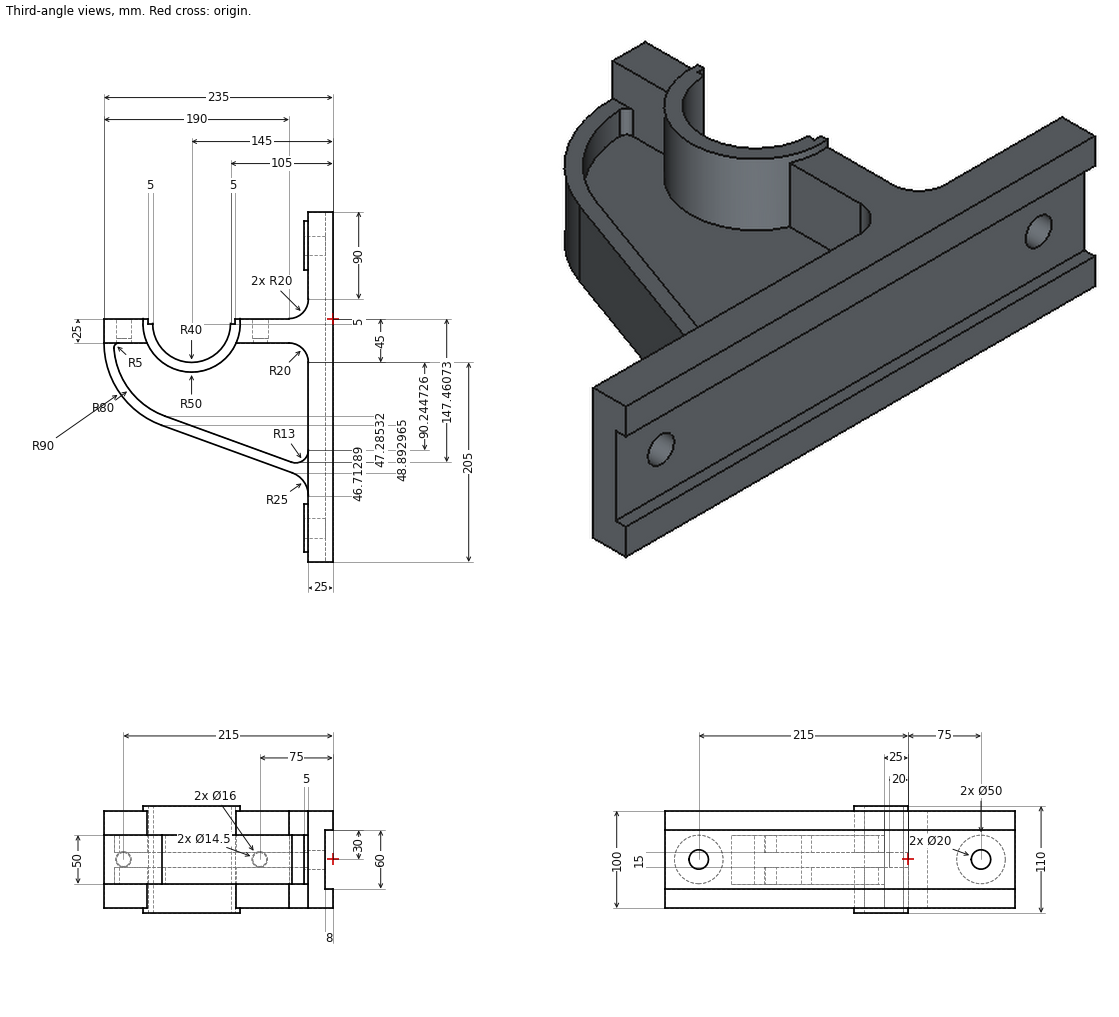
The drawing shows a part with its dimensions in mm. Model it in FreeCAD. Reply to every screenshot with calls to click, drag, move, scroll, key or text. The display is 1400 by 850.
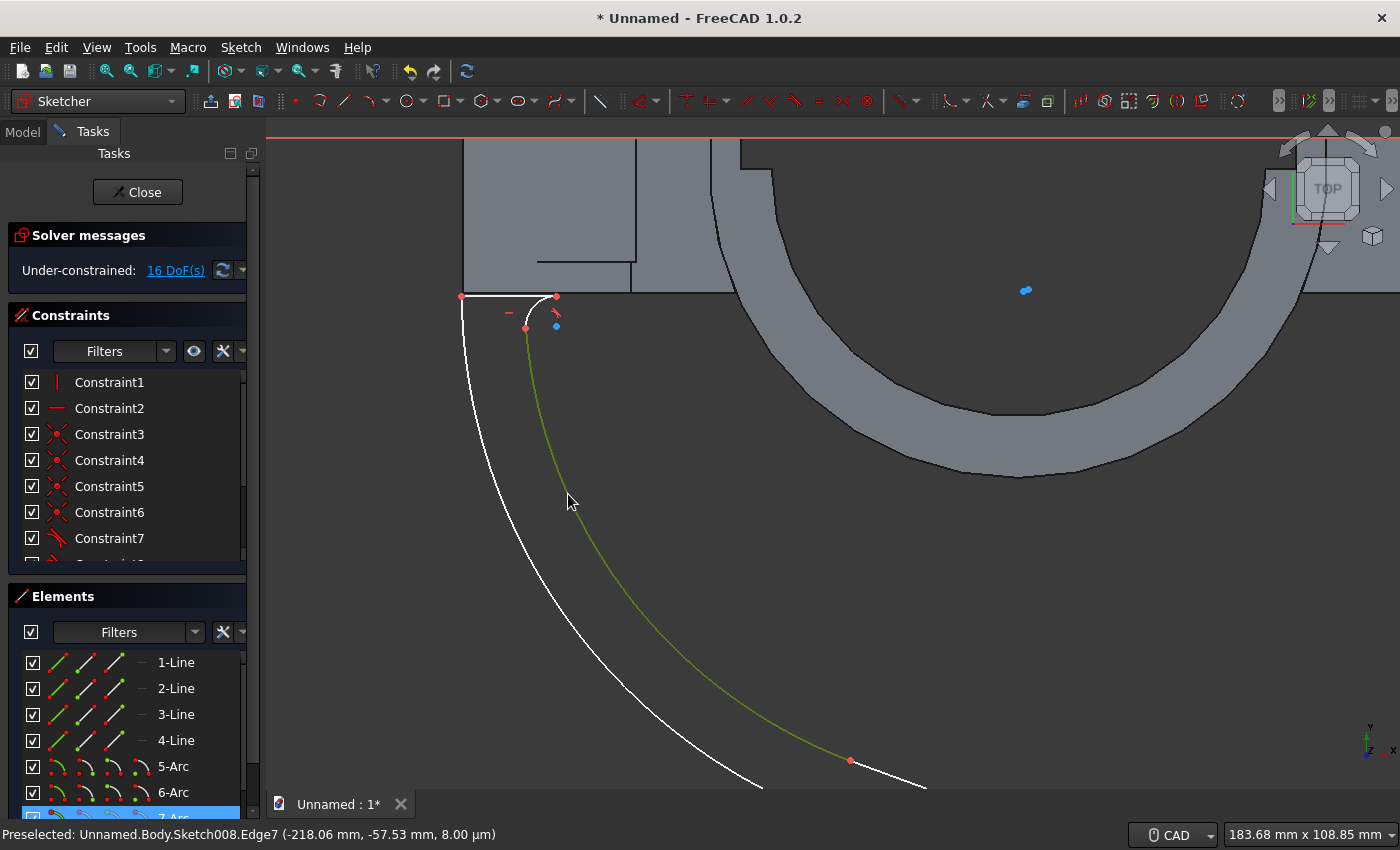
click(529, 314)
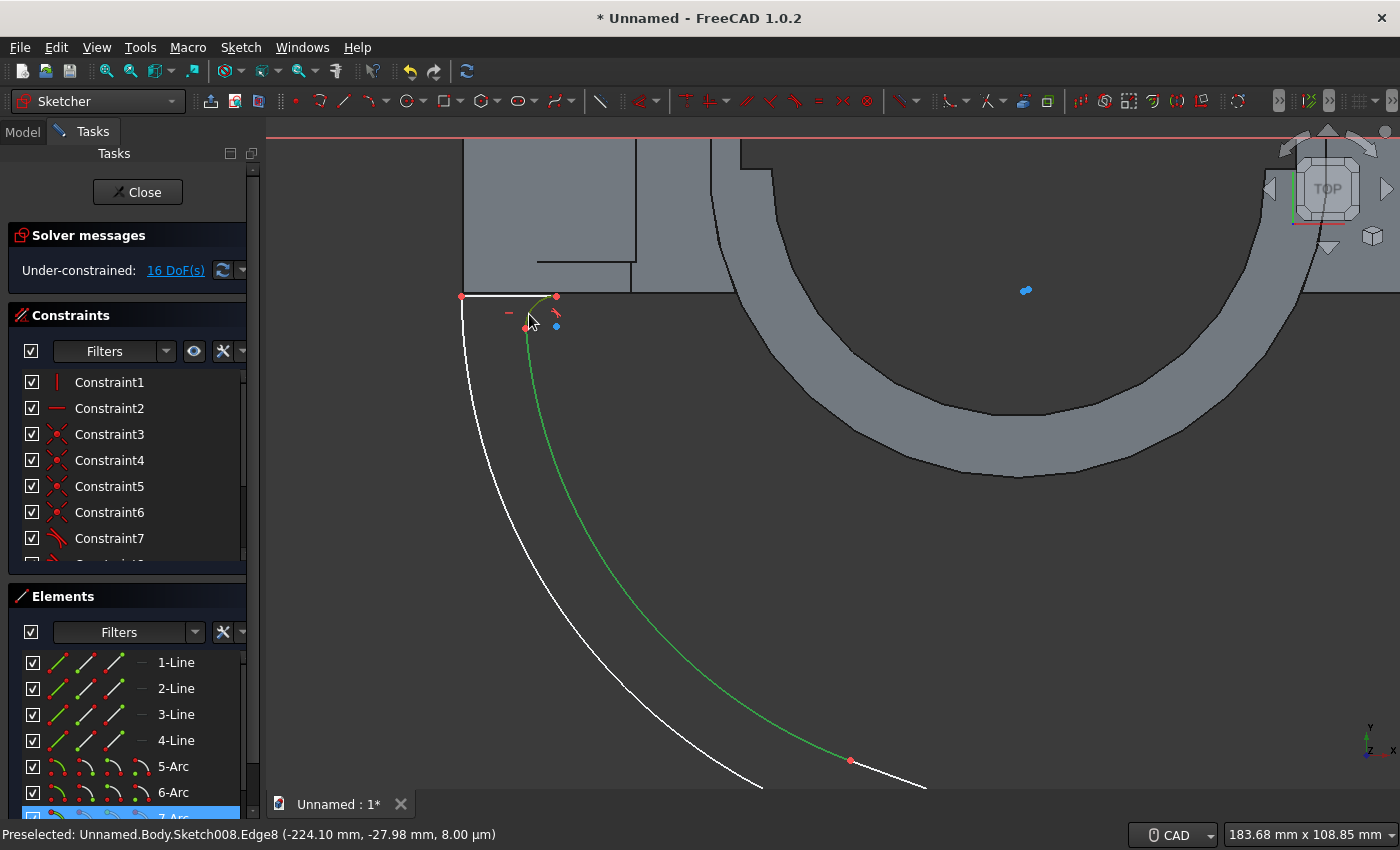
click(796, 102)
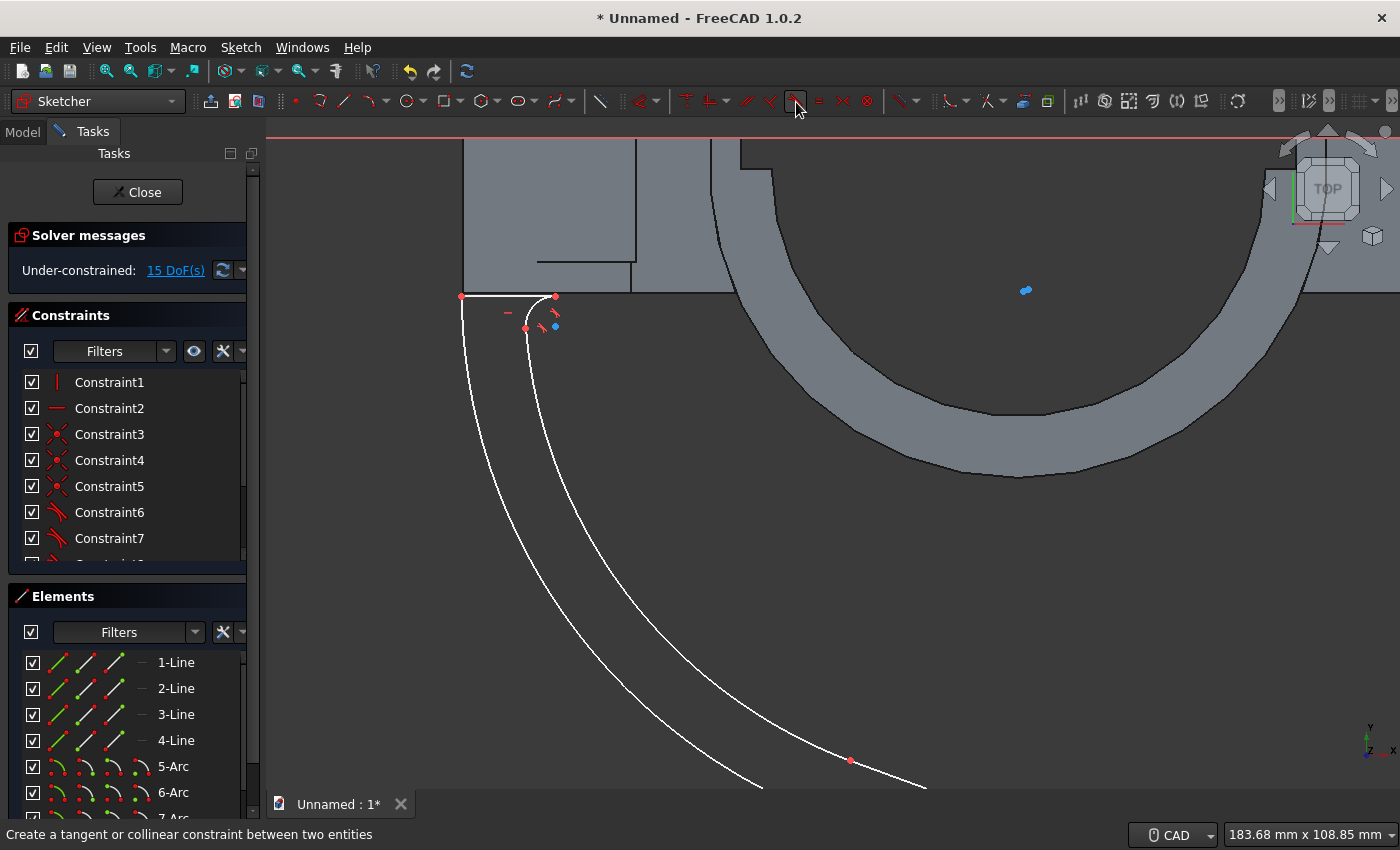
click(568, 494)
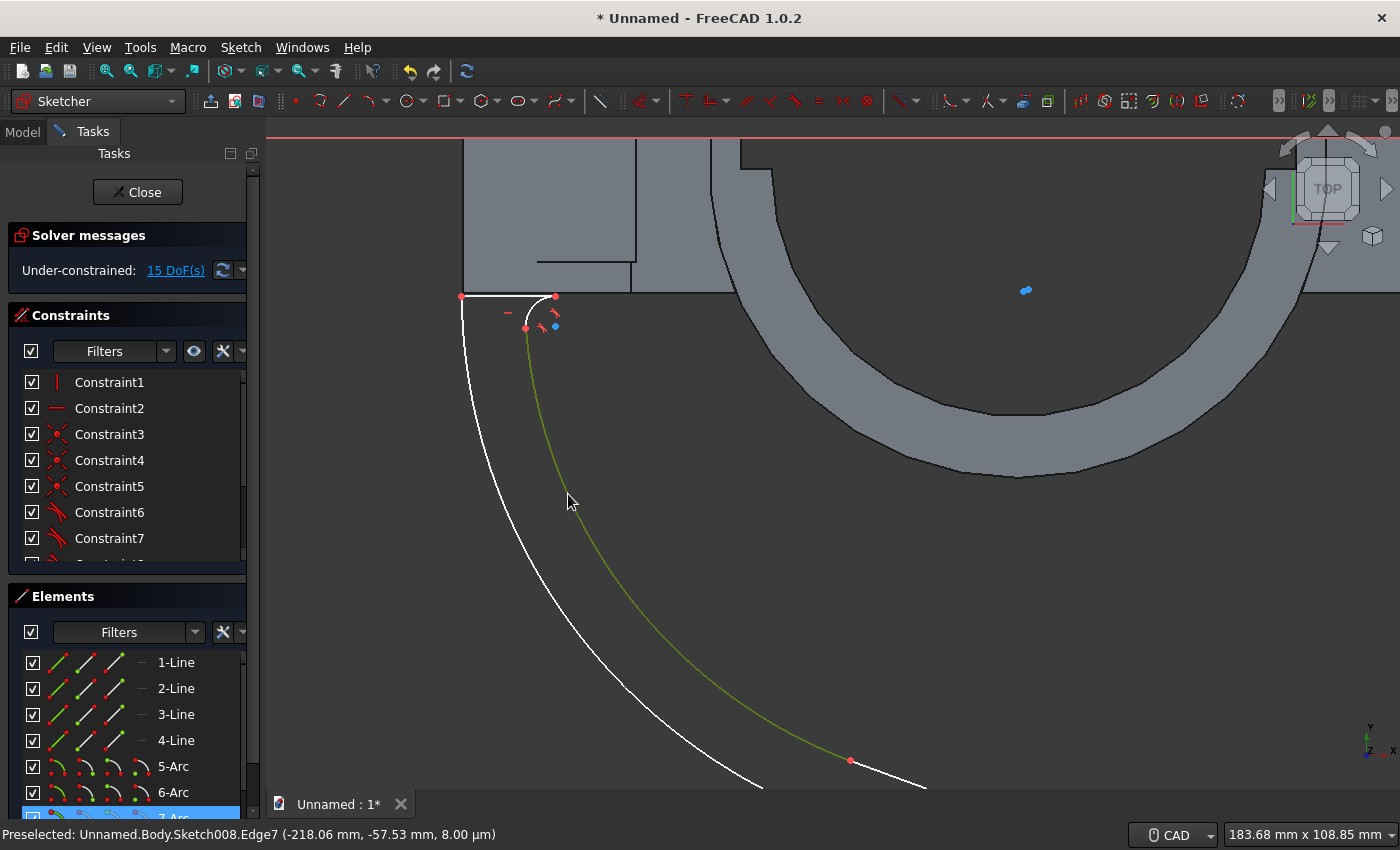
click(500, 495)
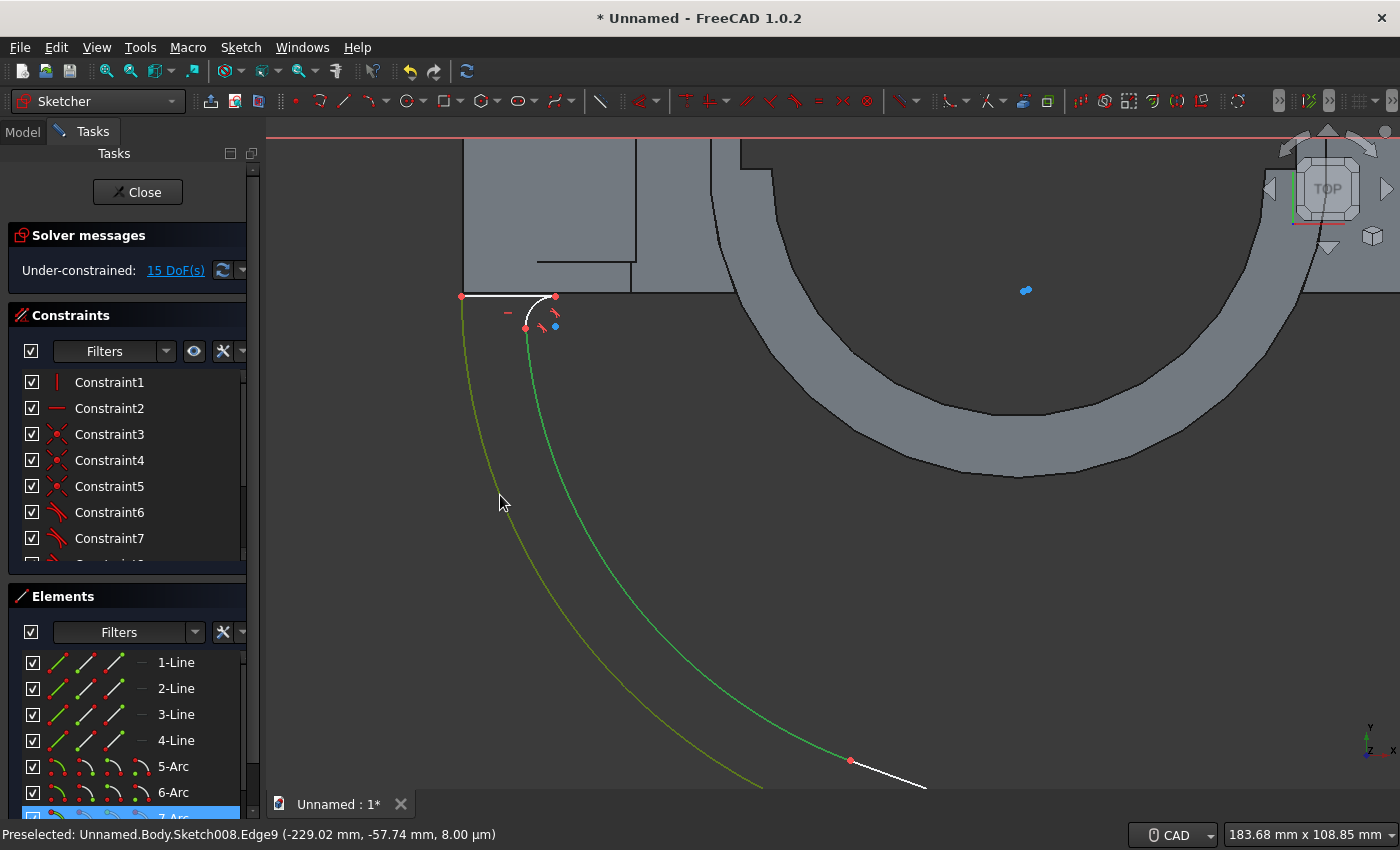
click(686, 102)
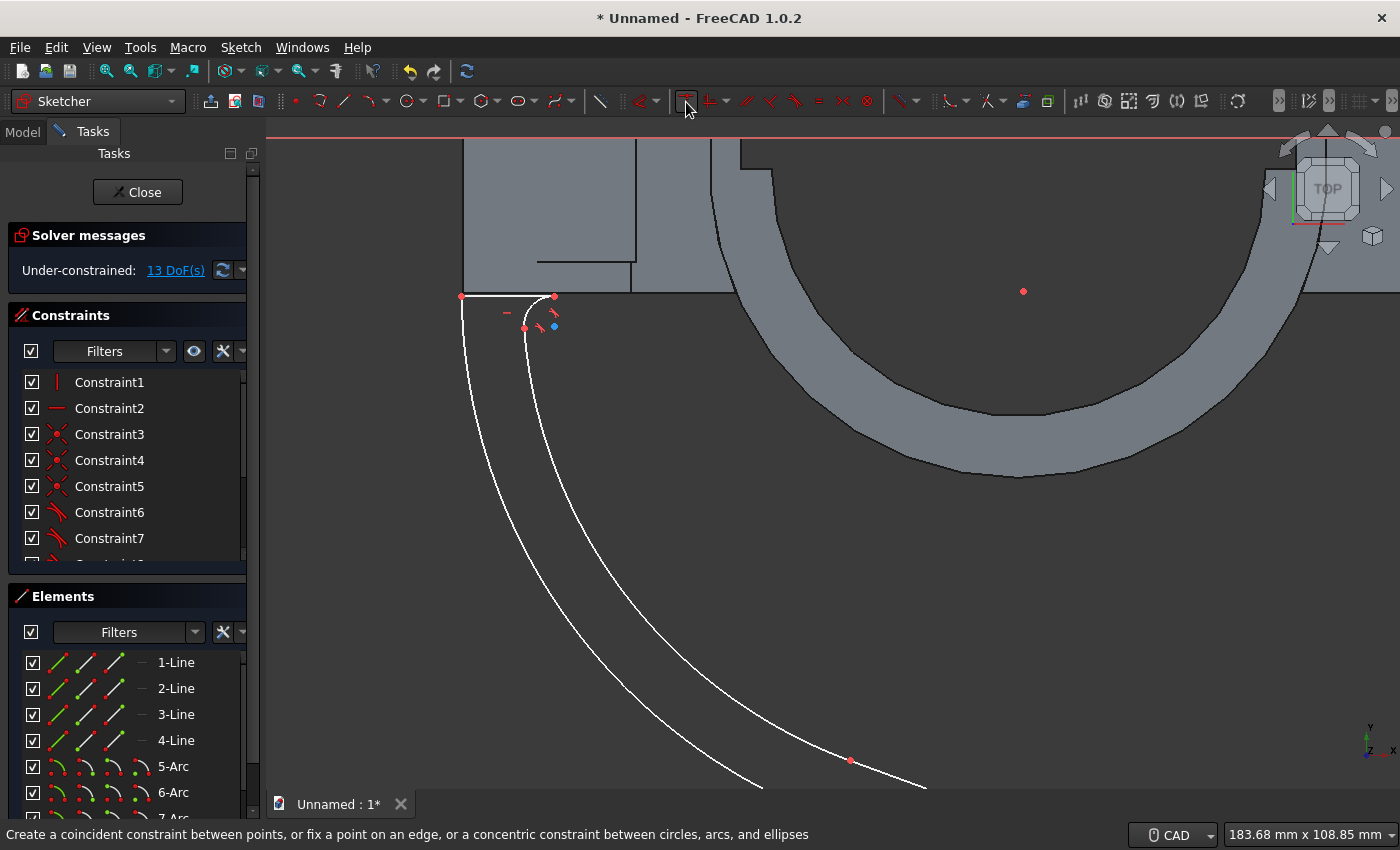
click(640, 102)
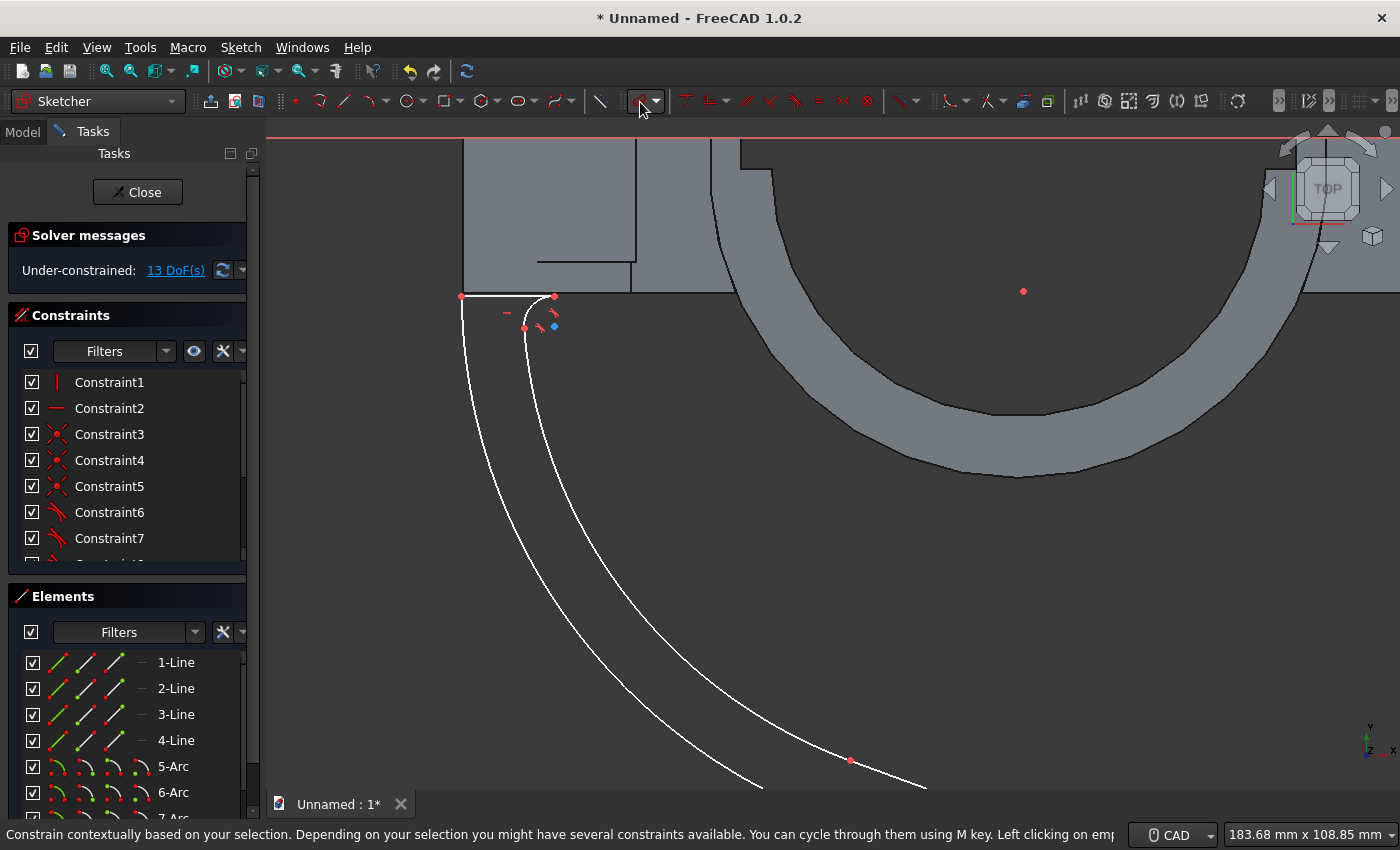
scroll(518, 309, down, 5)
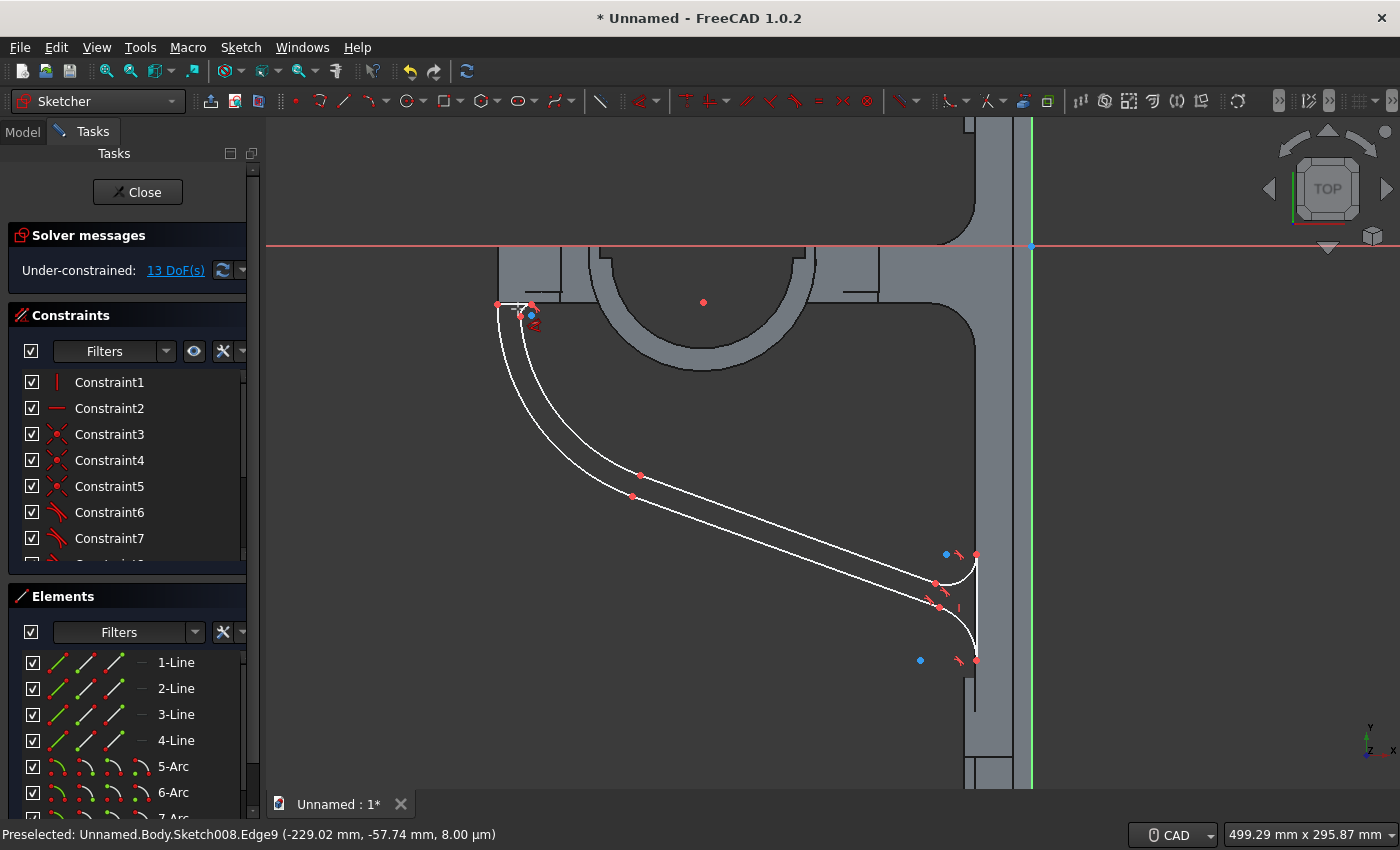
scroll(973, 640, up, 7)